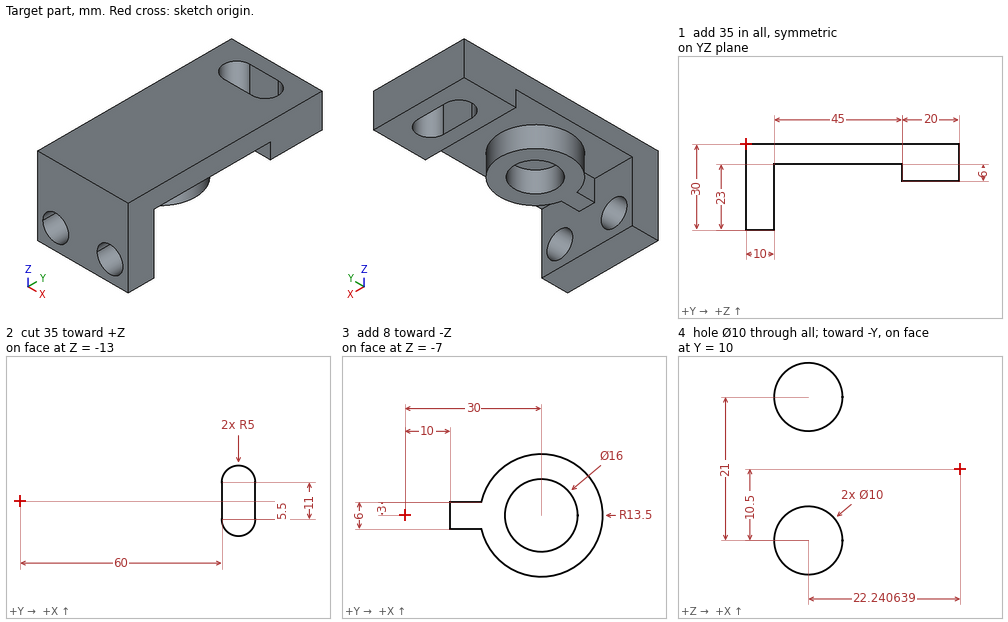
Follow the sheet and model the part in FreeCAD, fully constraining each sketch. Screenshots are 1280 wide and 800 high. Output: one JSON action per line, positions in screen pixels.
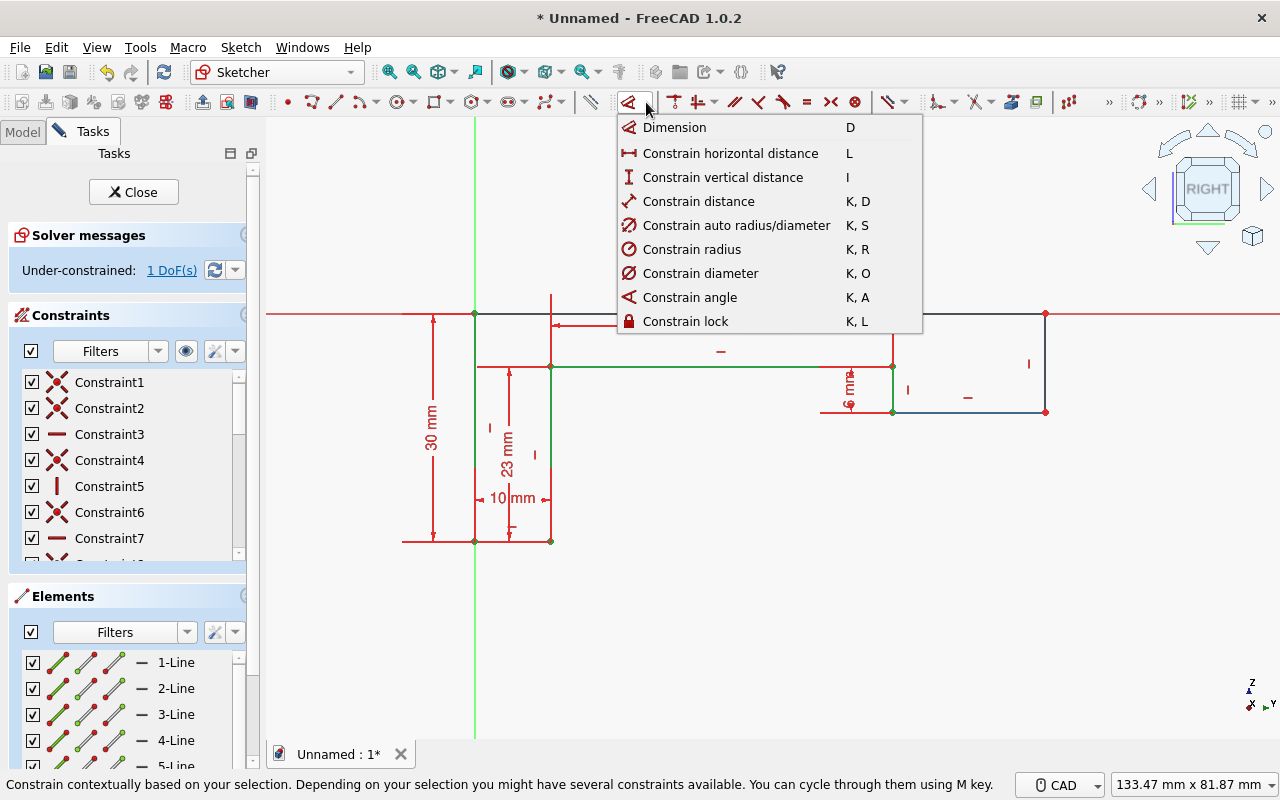
{"action": "left_click", "coordinate": [770, 153]}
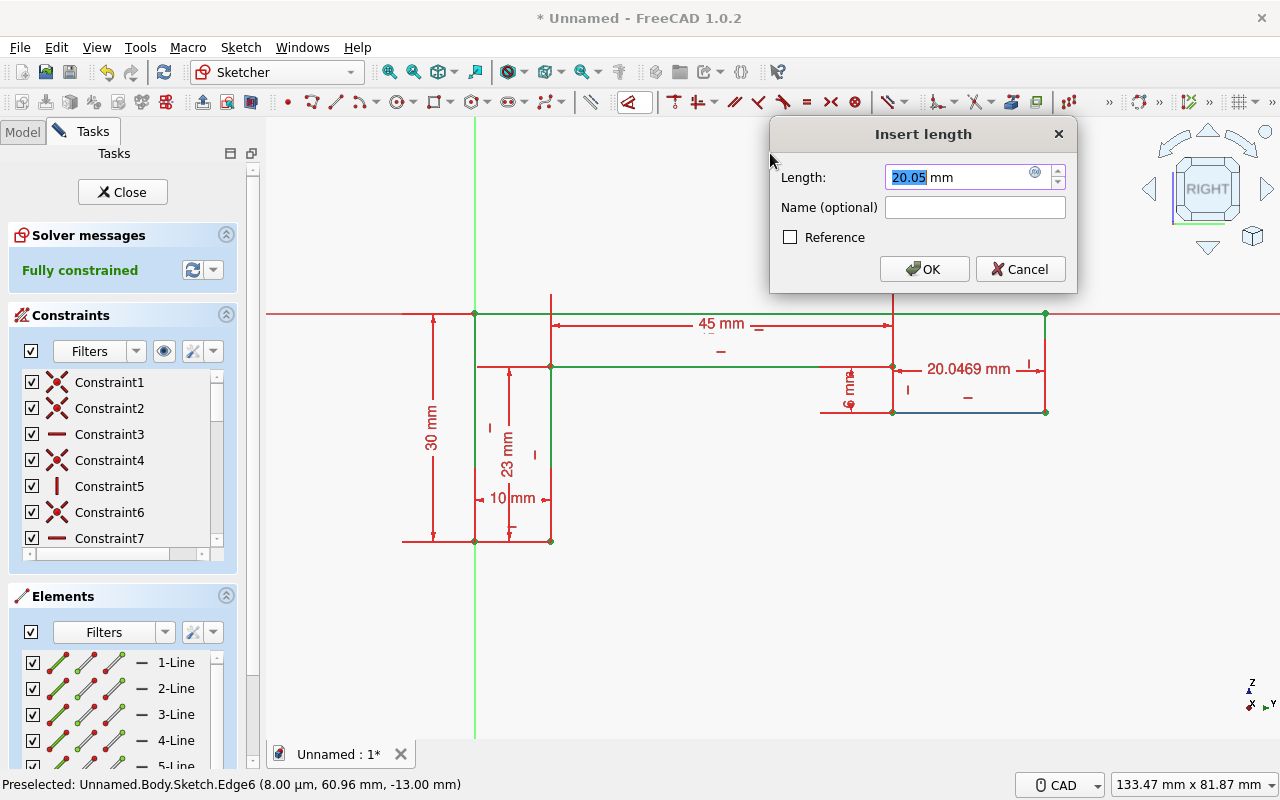
{"action": "type", "text": "20"}
{"action": "key", "text": "Return"}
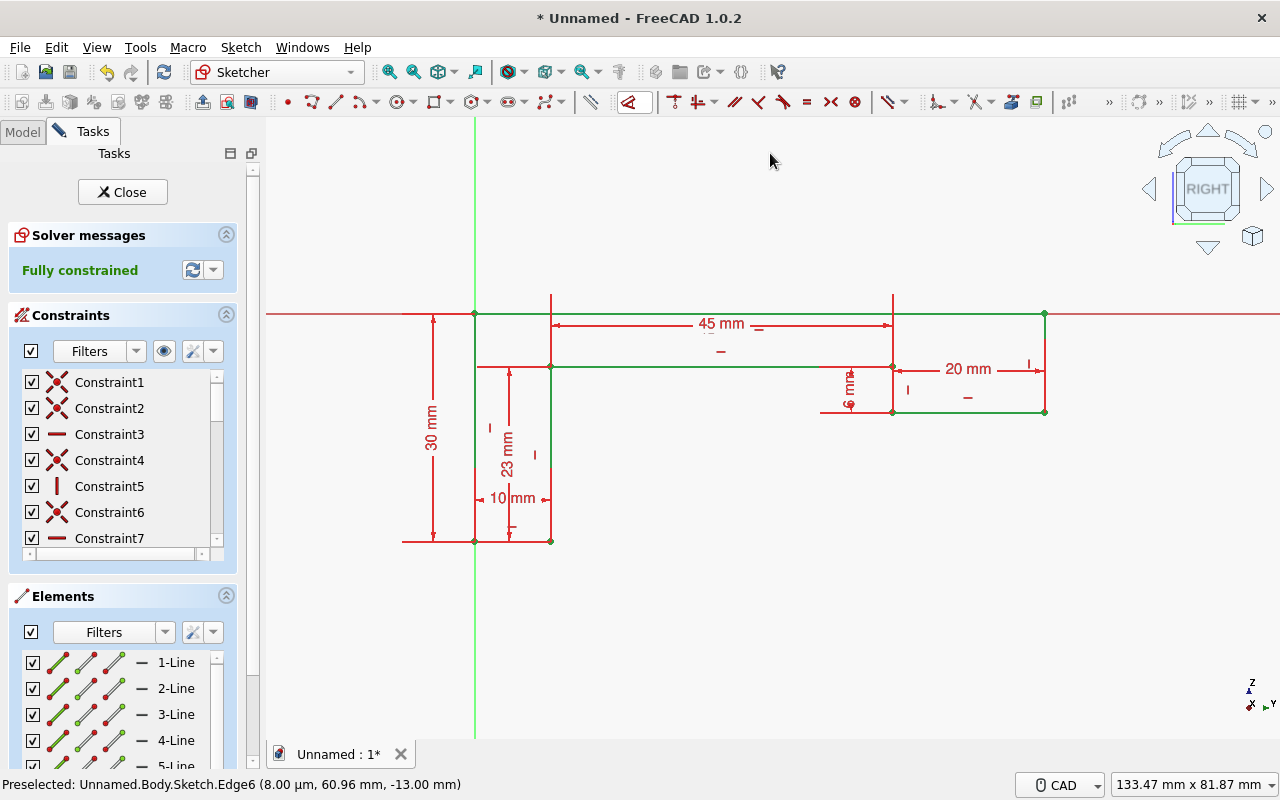
{"action": "left_click", "coordinate": [123, 192]}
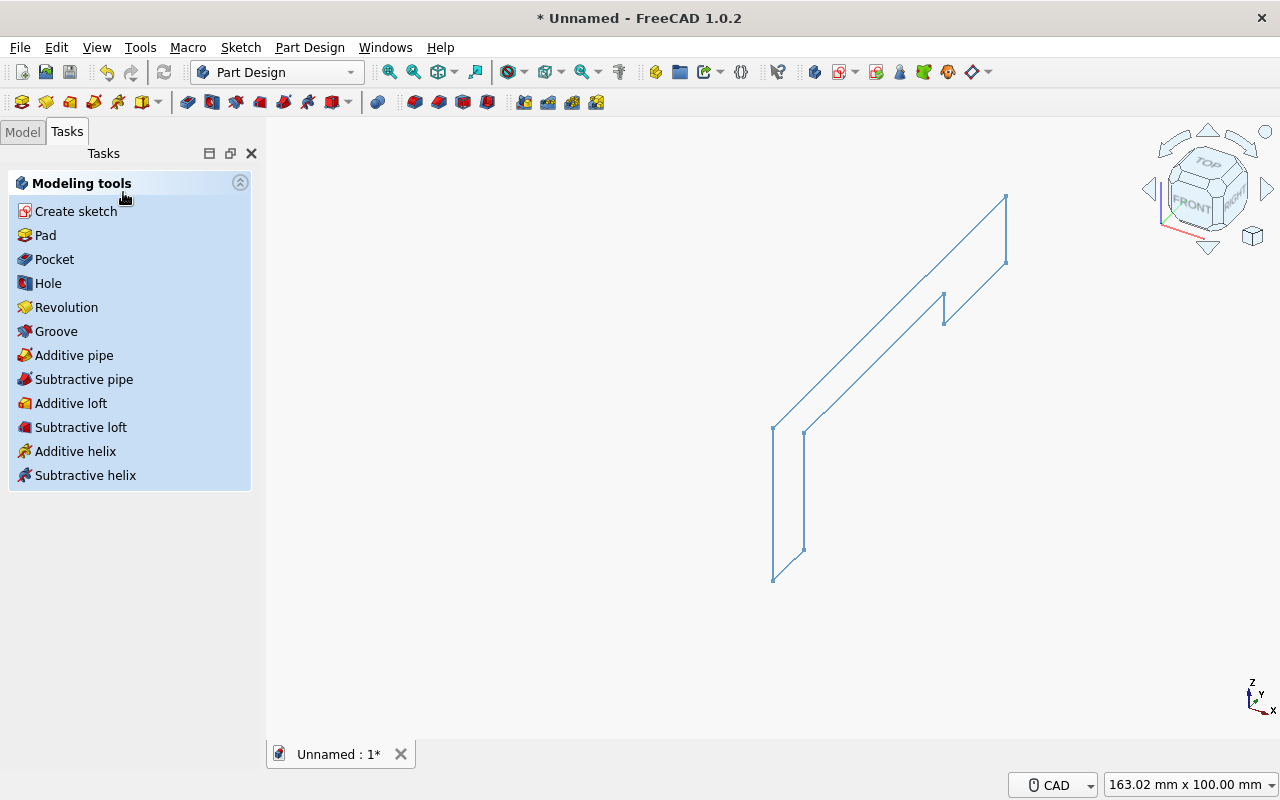
{"action": "left_click", "coordinate": [22, 102]}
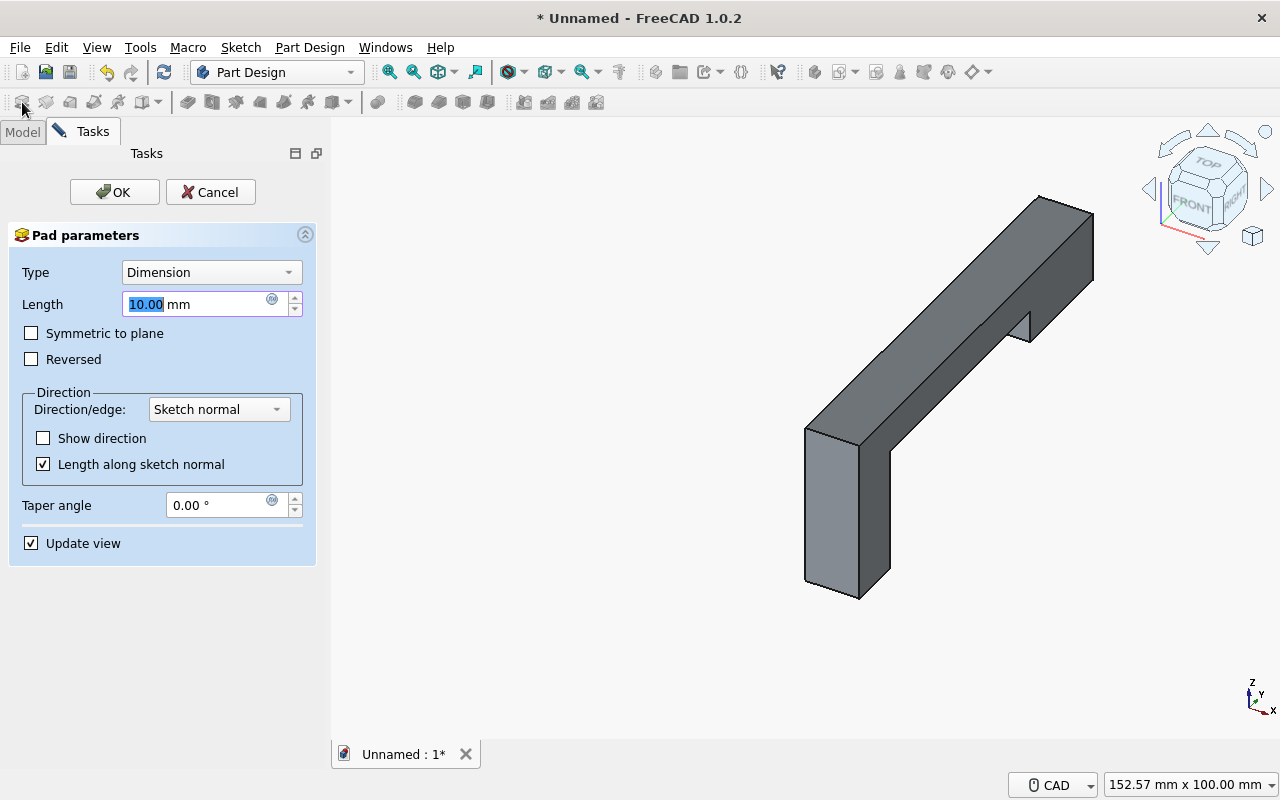
{"action": "type", "text": "35"}
{"action": "key", "text": "Tab"}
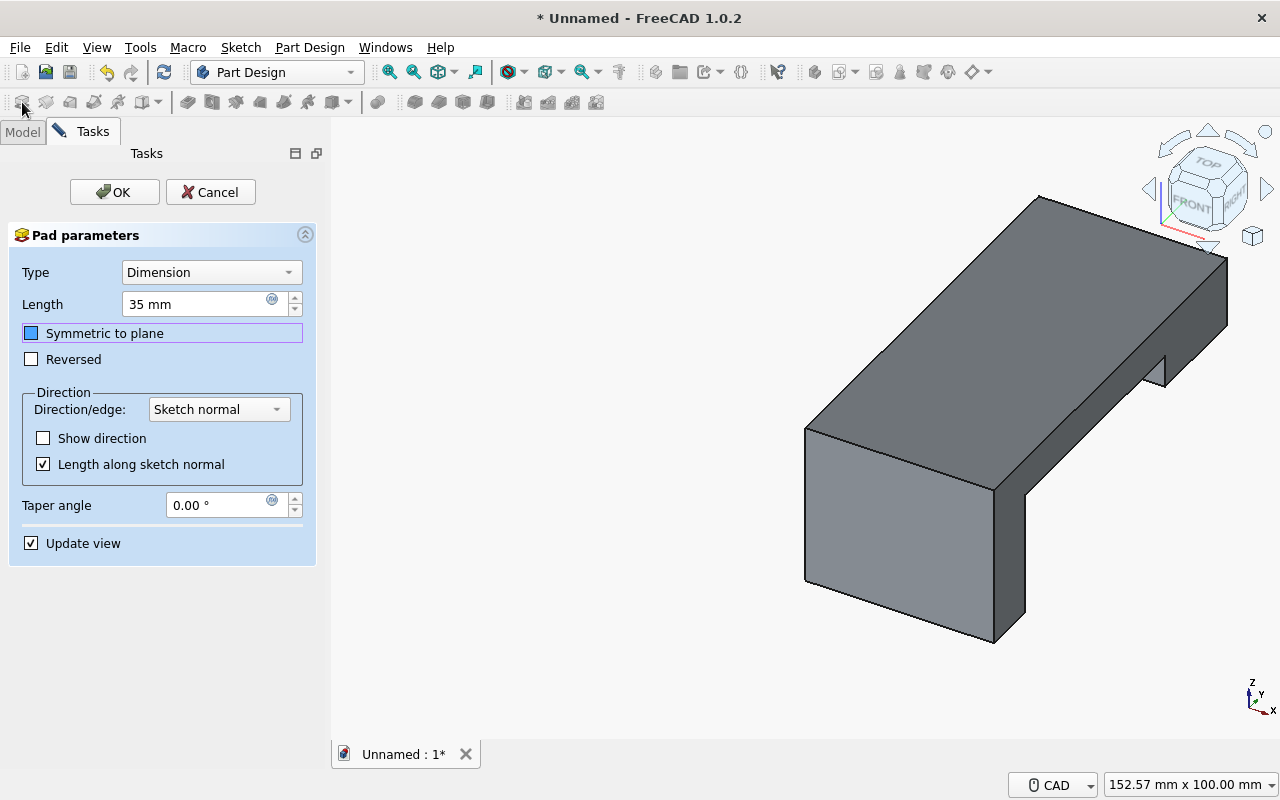
{"action": "left_click", "coordinate": [30, 333]}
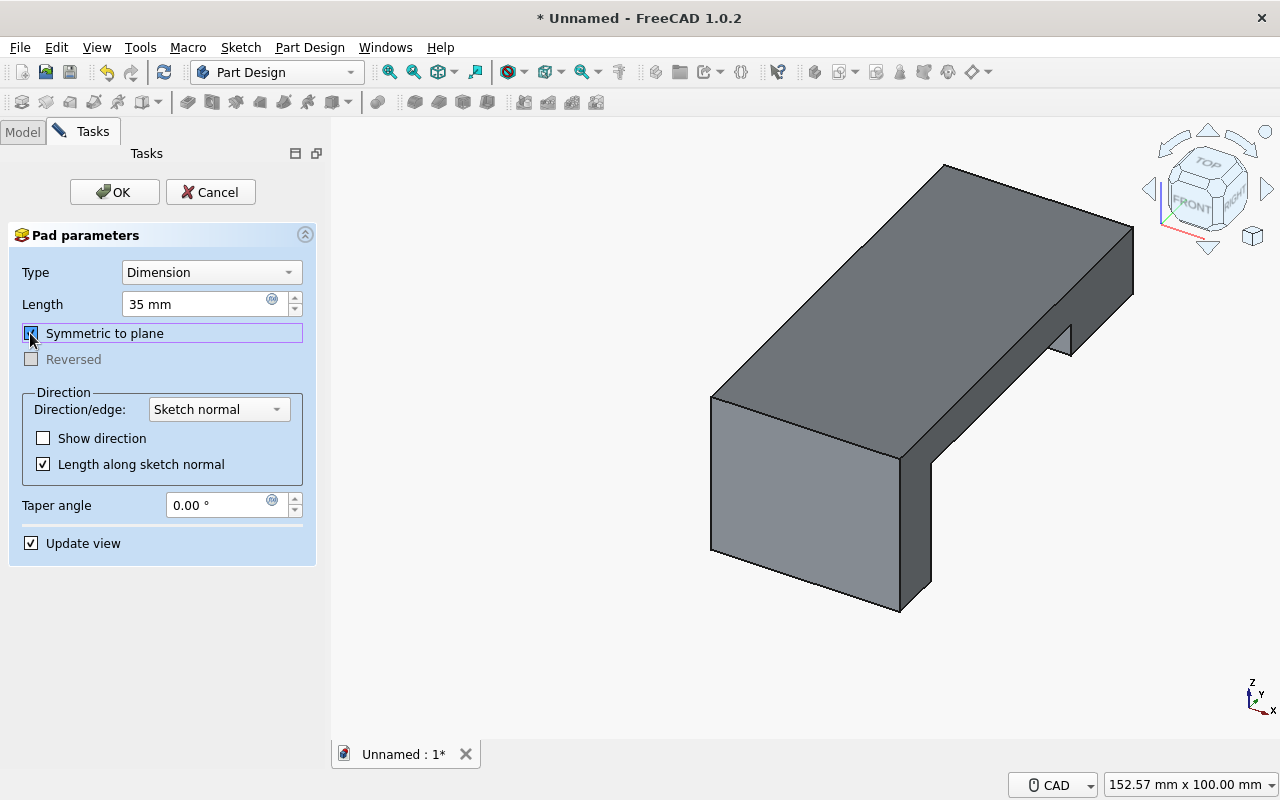
{"action": "left_click", "coordinate": [115, 192]}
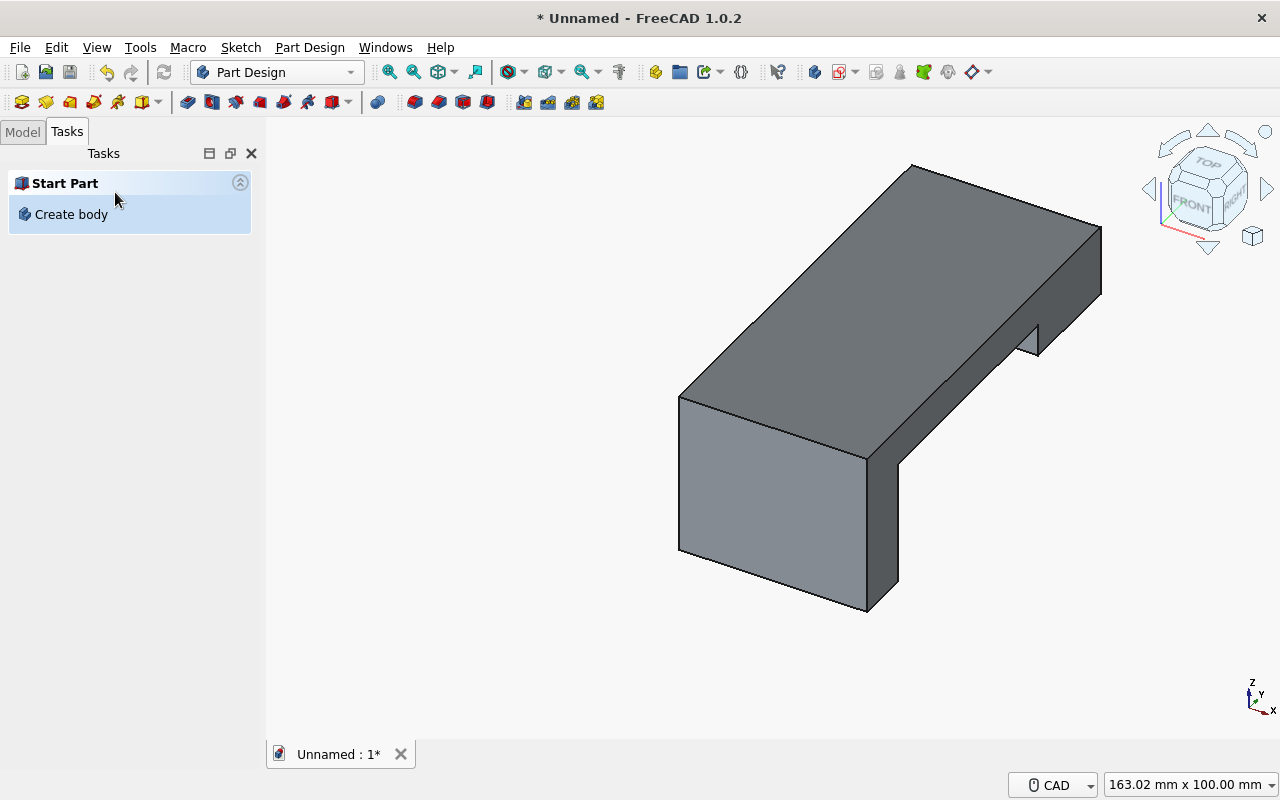
{"action": "key", "text": "5"}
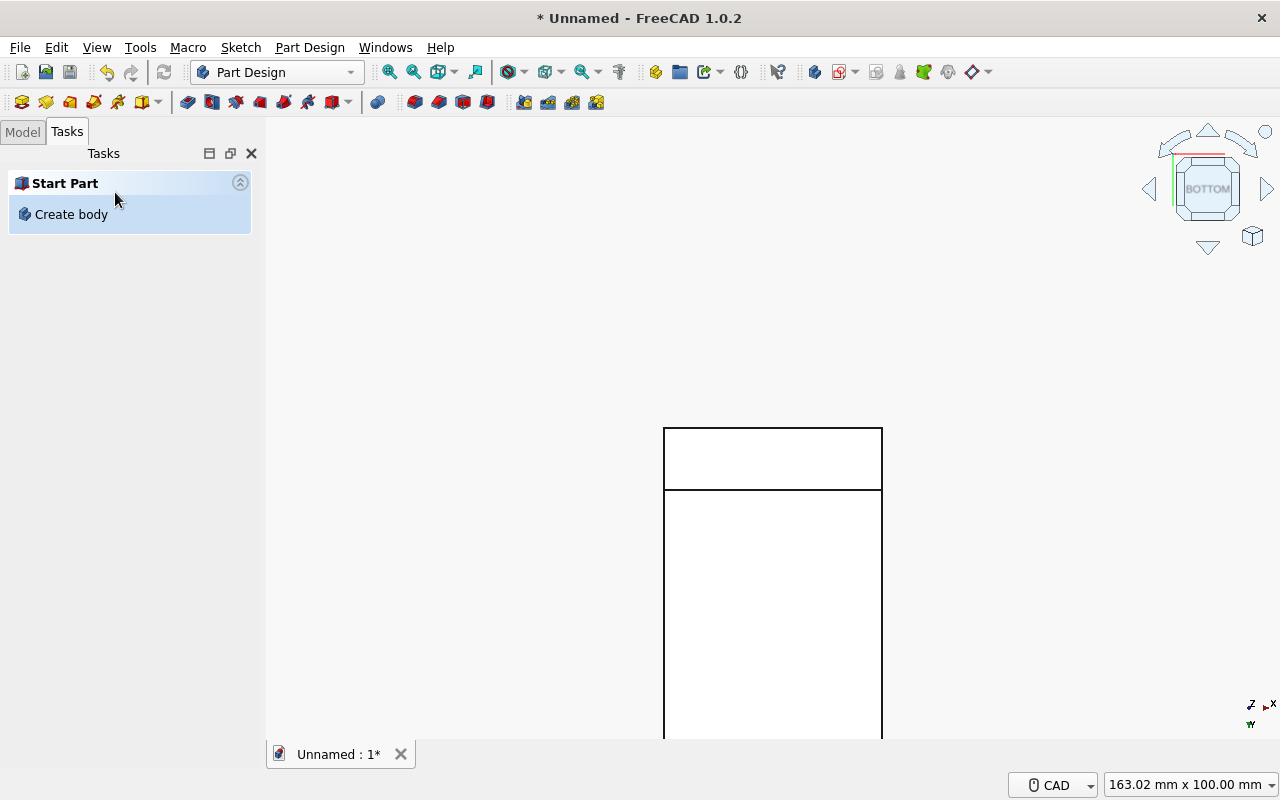
{"action": "left_click", "coordinate": [390, 72]}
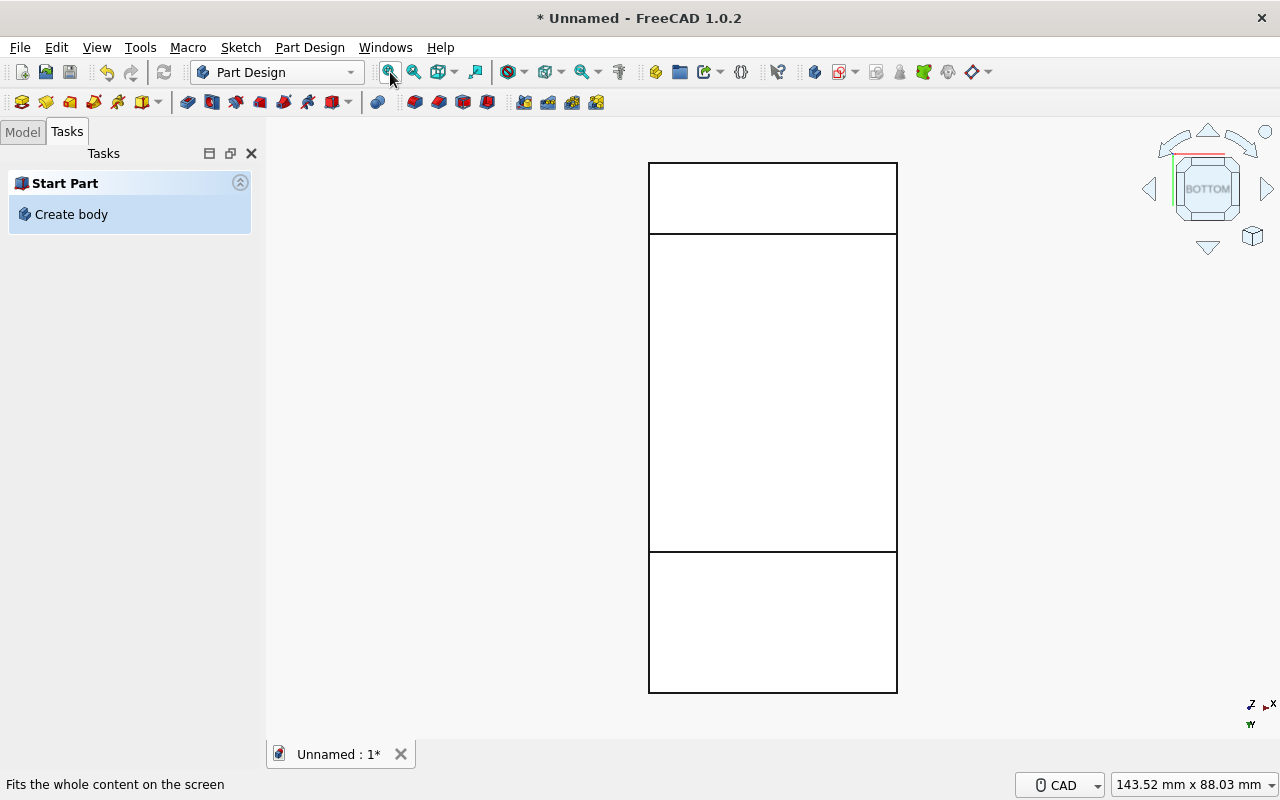
{"action": "left_click", "coordinate": [808, 621]}